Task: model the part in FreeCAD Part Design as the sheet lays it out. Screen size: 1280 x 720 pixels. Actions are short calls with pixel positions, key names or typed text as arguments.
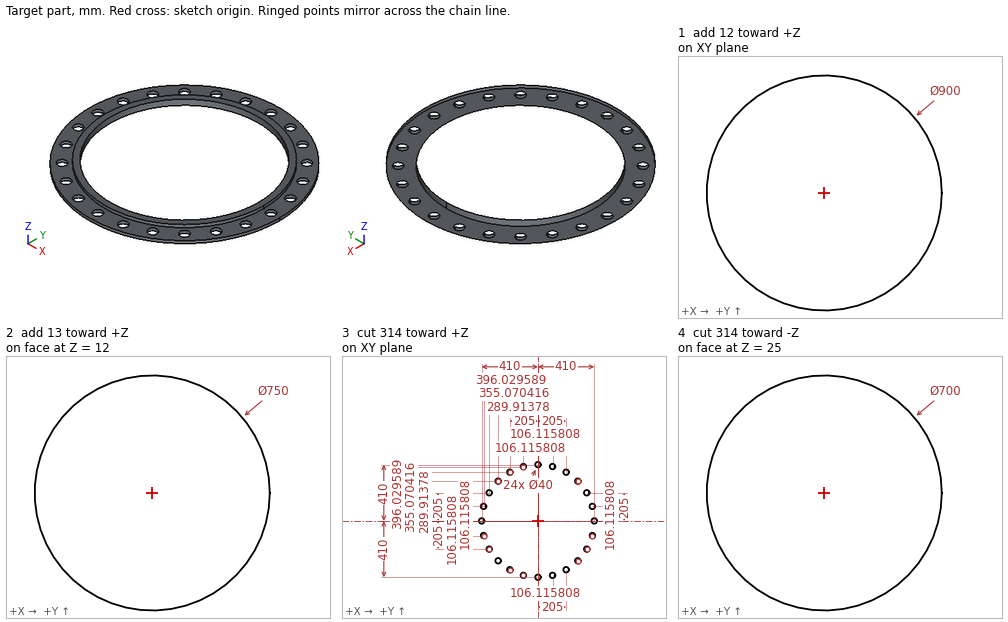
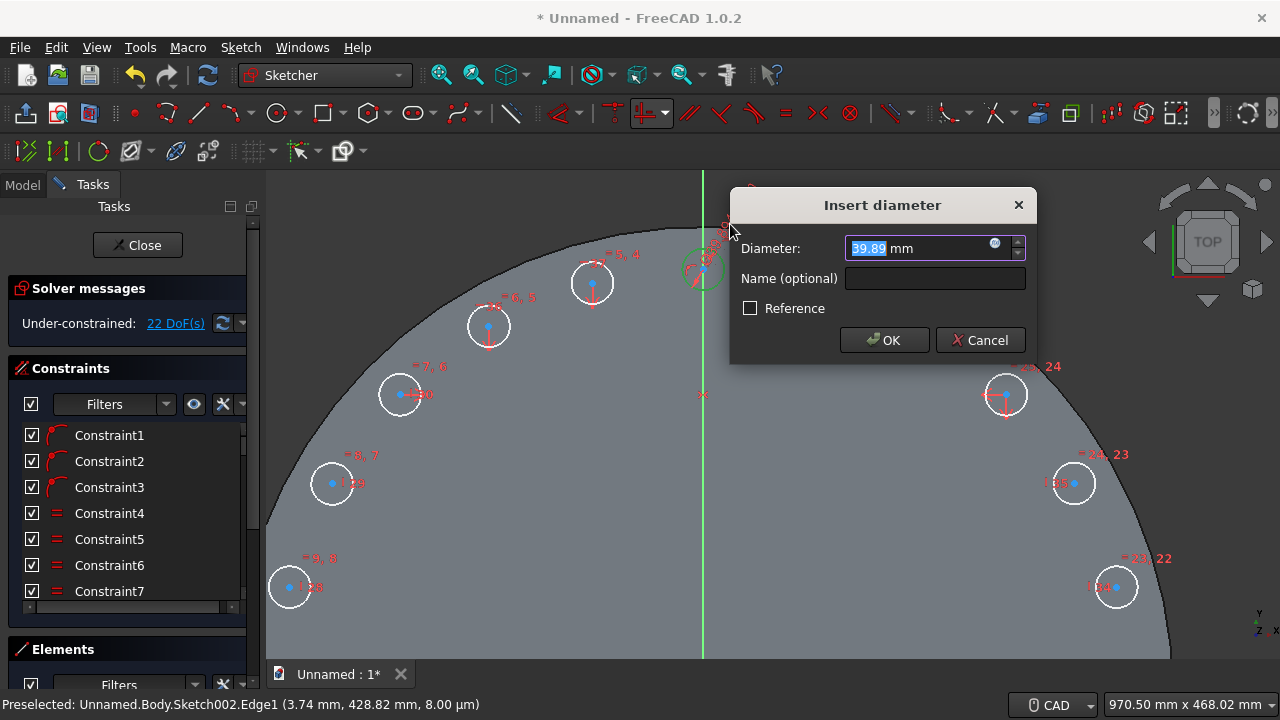
text(40)
key(Return)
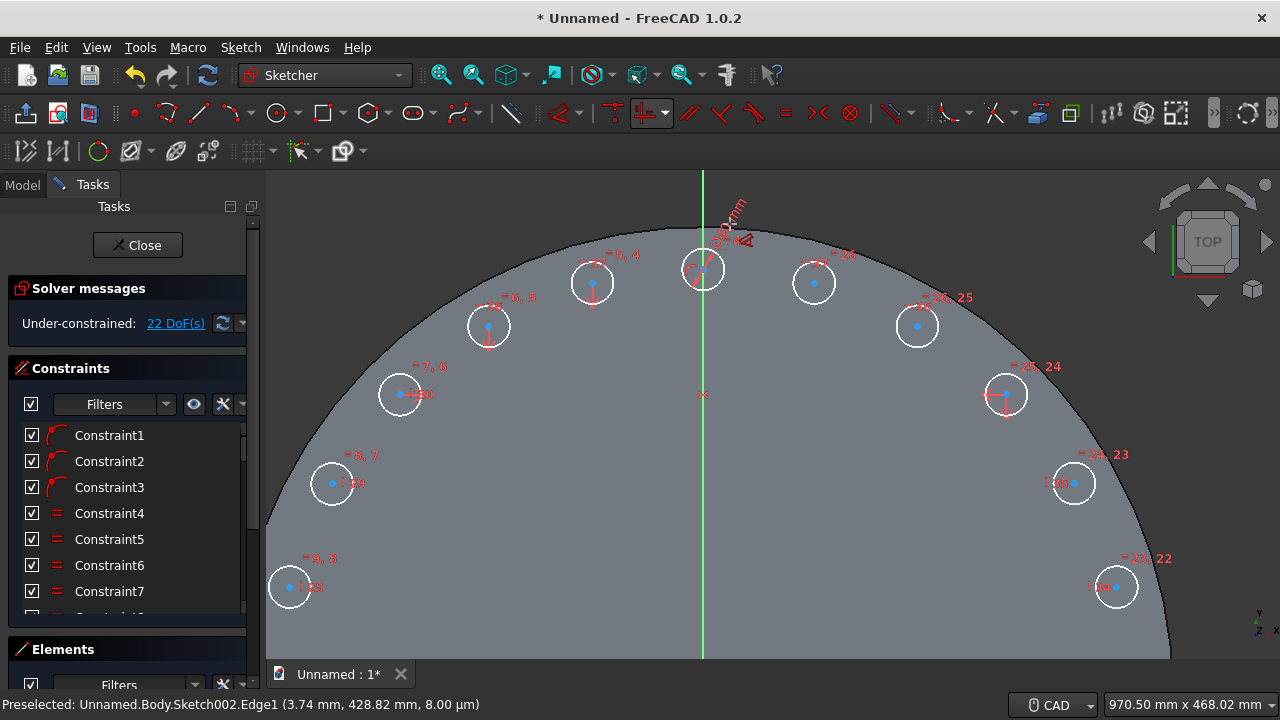
click(703, 269)
click(737, 450)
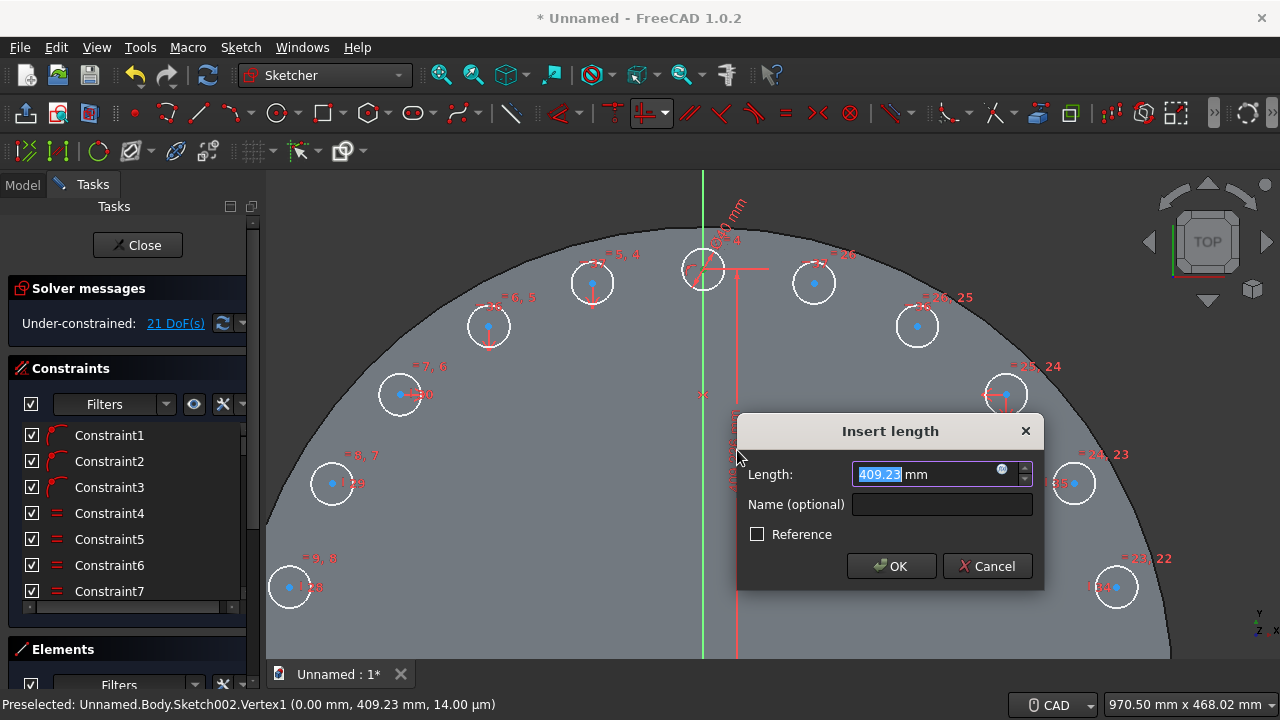
text(410)
key(Return)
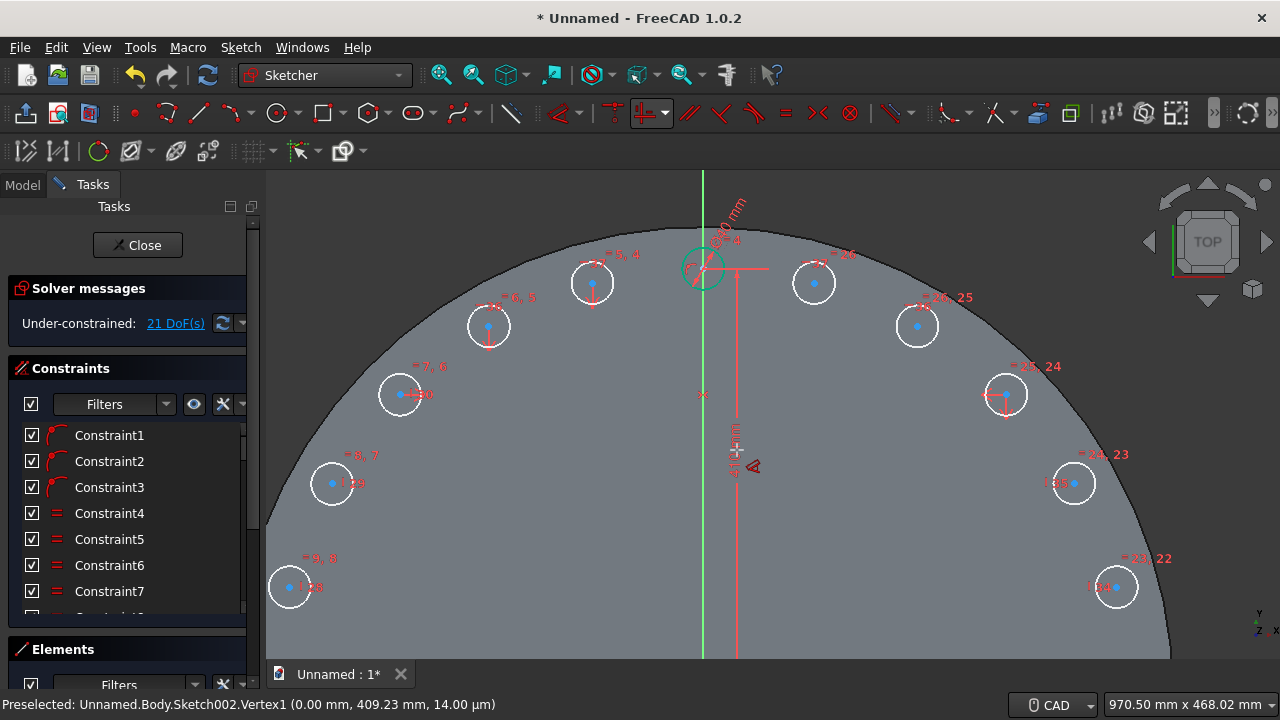
click(489, 326)
click(547, 292)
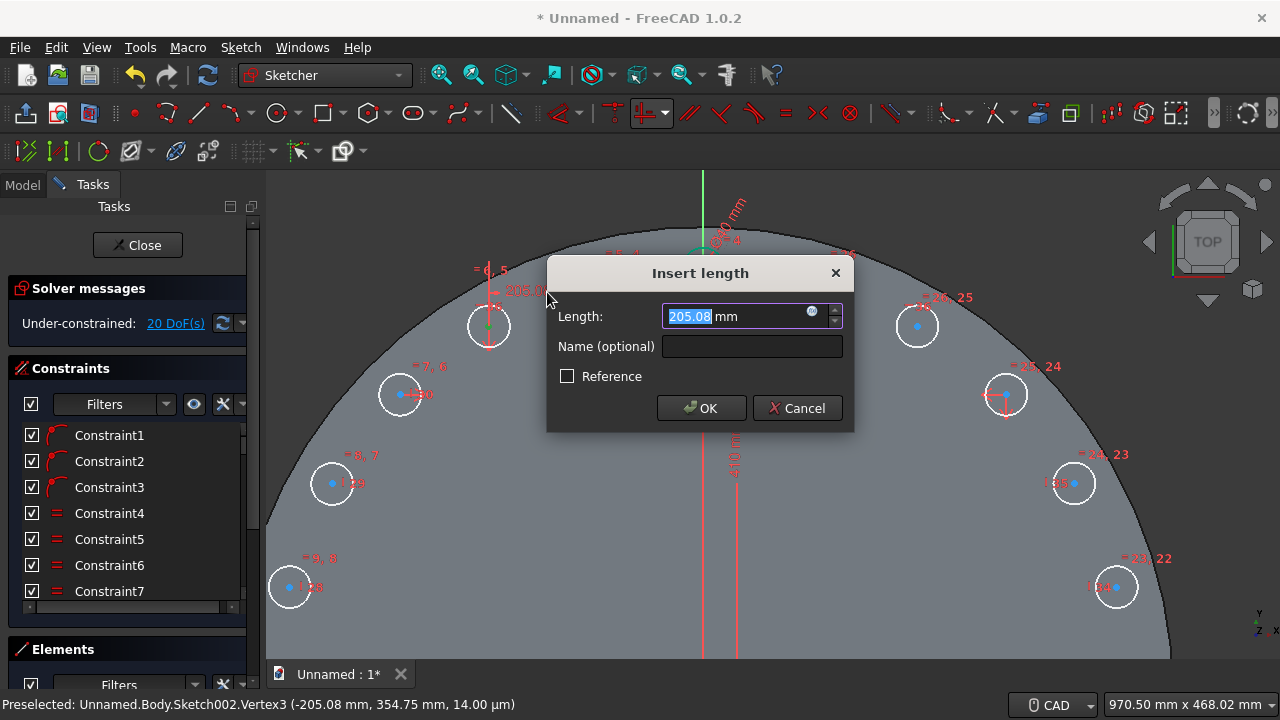
text(205)
key(Return)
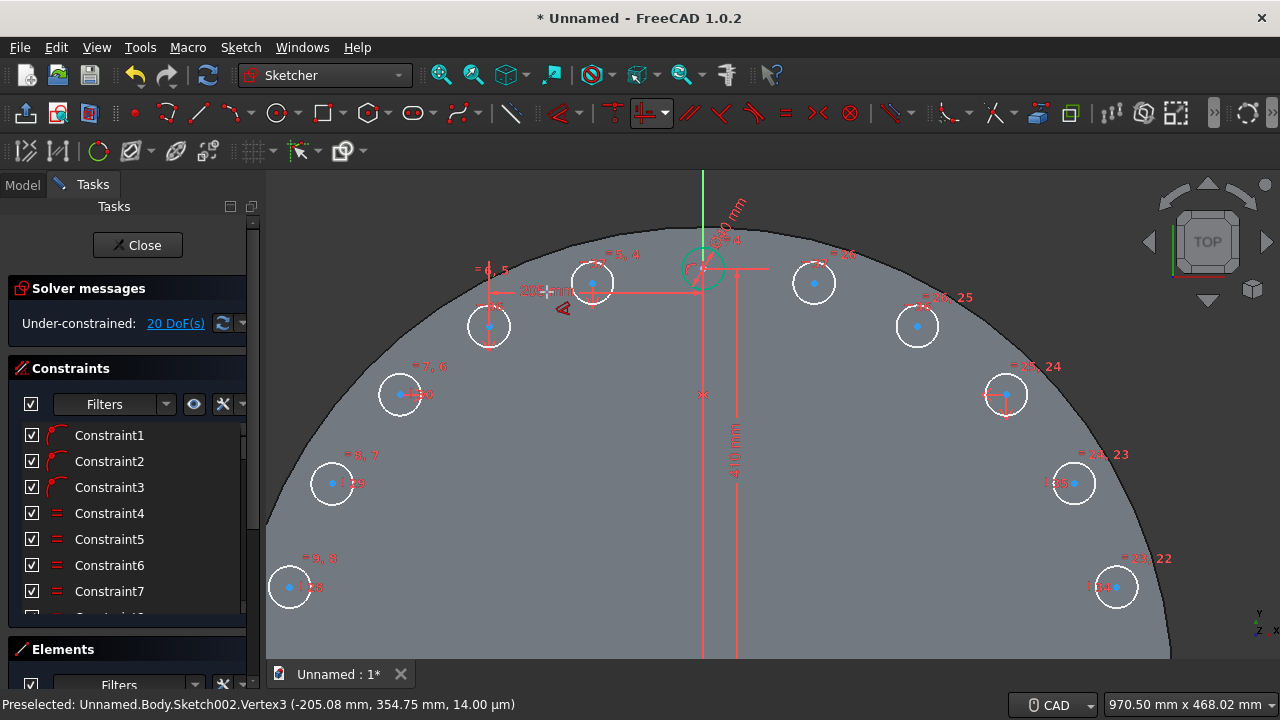
click(332, 484)
click(298, 524)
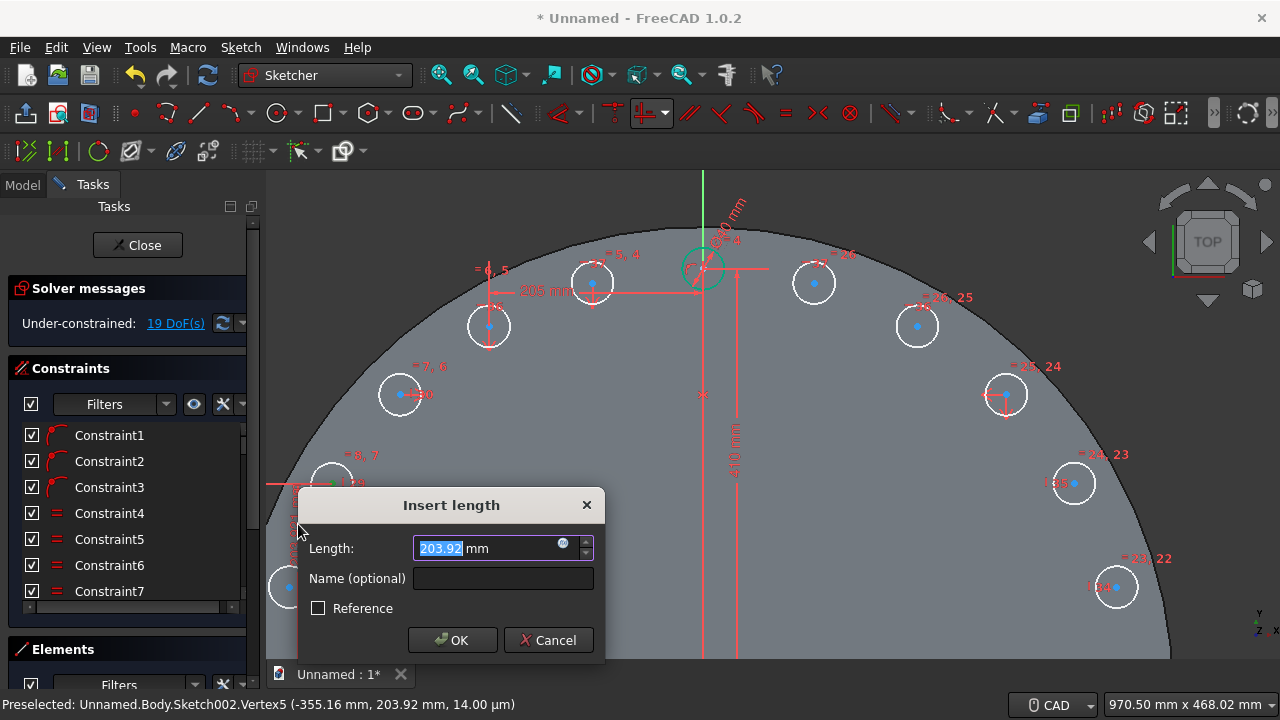
text(205)
key(Return)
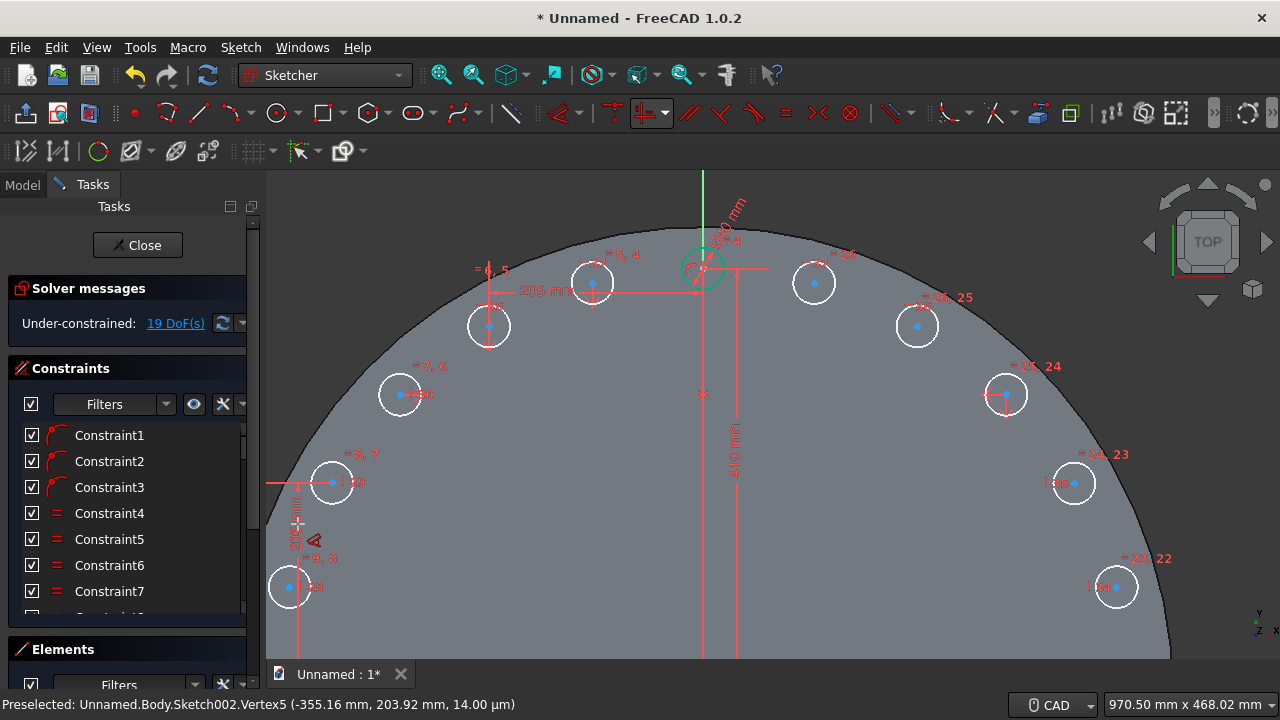
scroll(705, 250, down, 5)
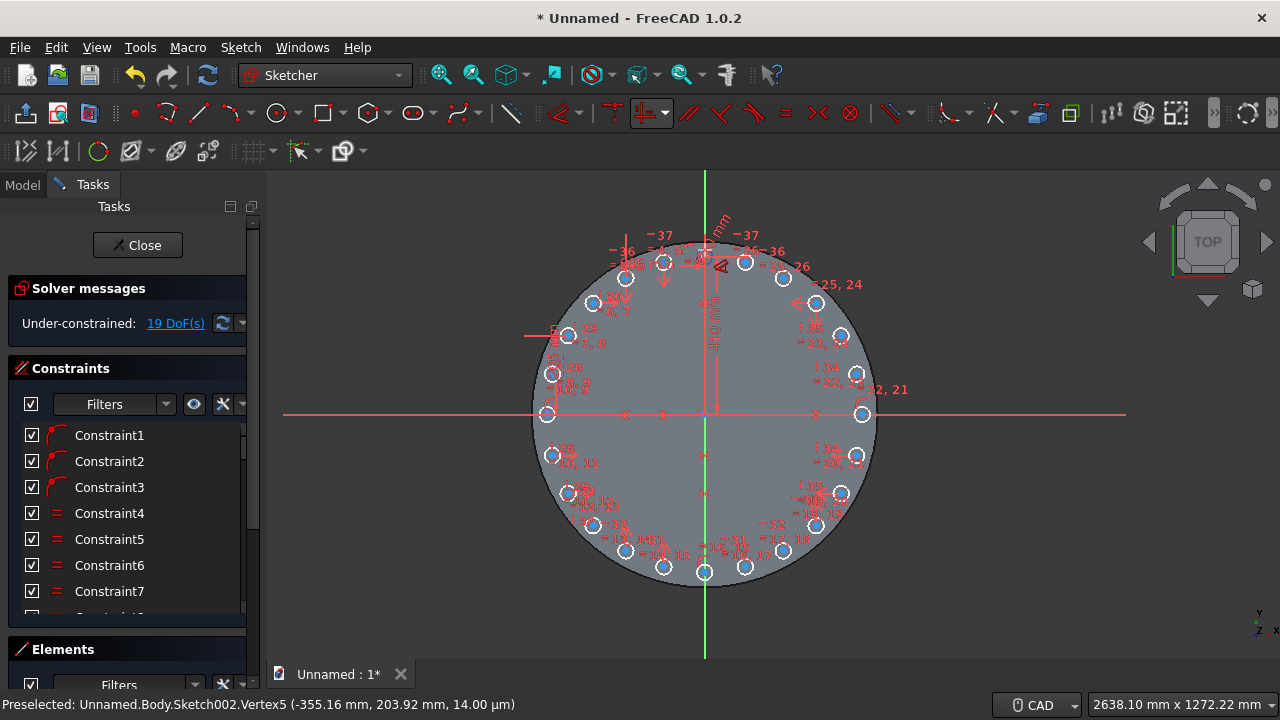
click(547, 415)
click(626, 449)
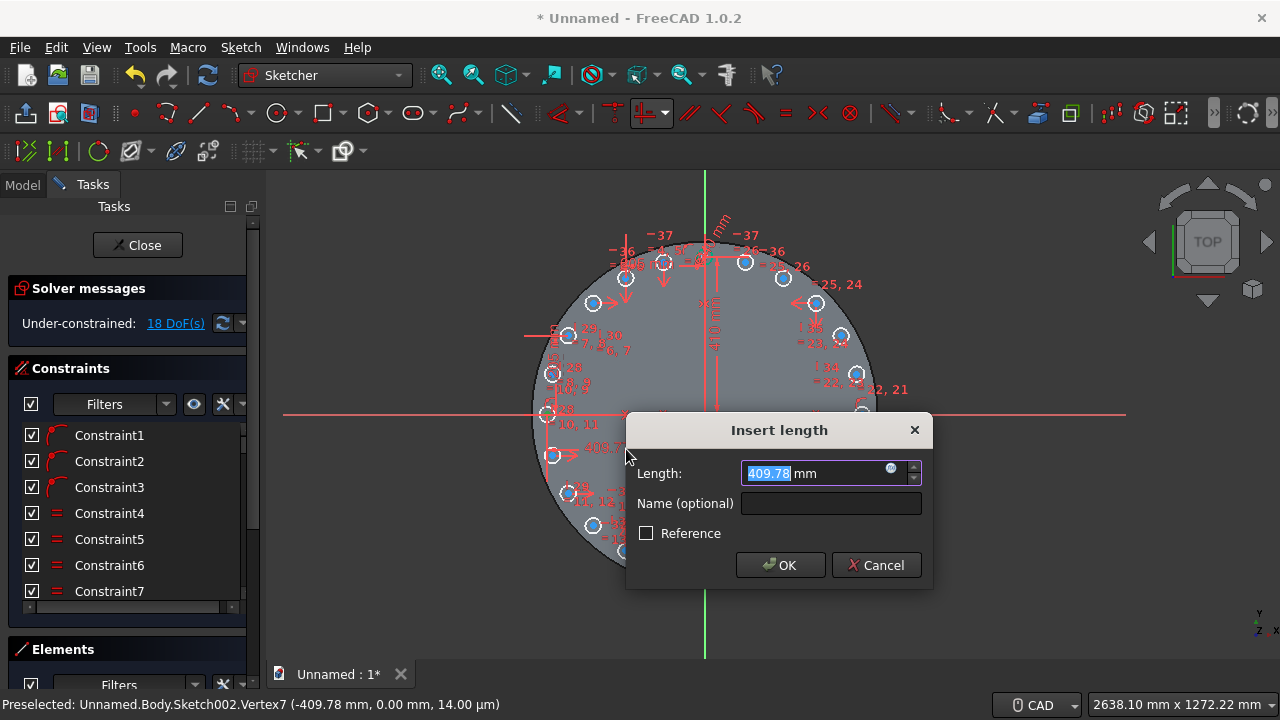
text(410)
key(Return)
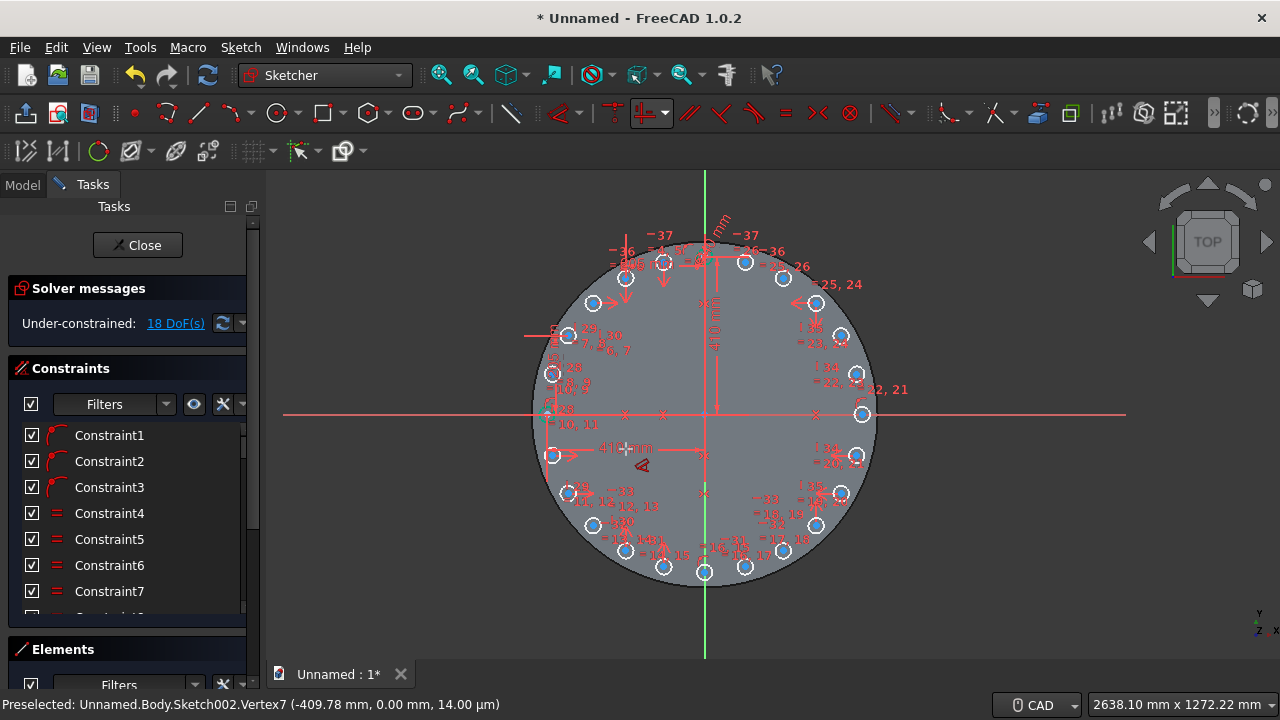
click(568, 494)
click(534, 436)